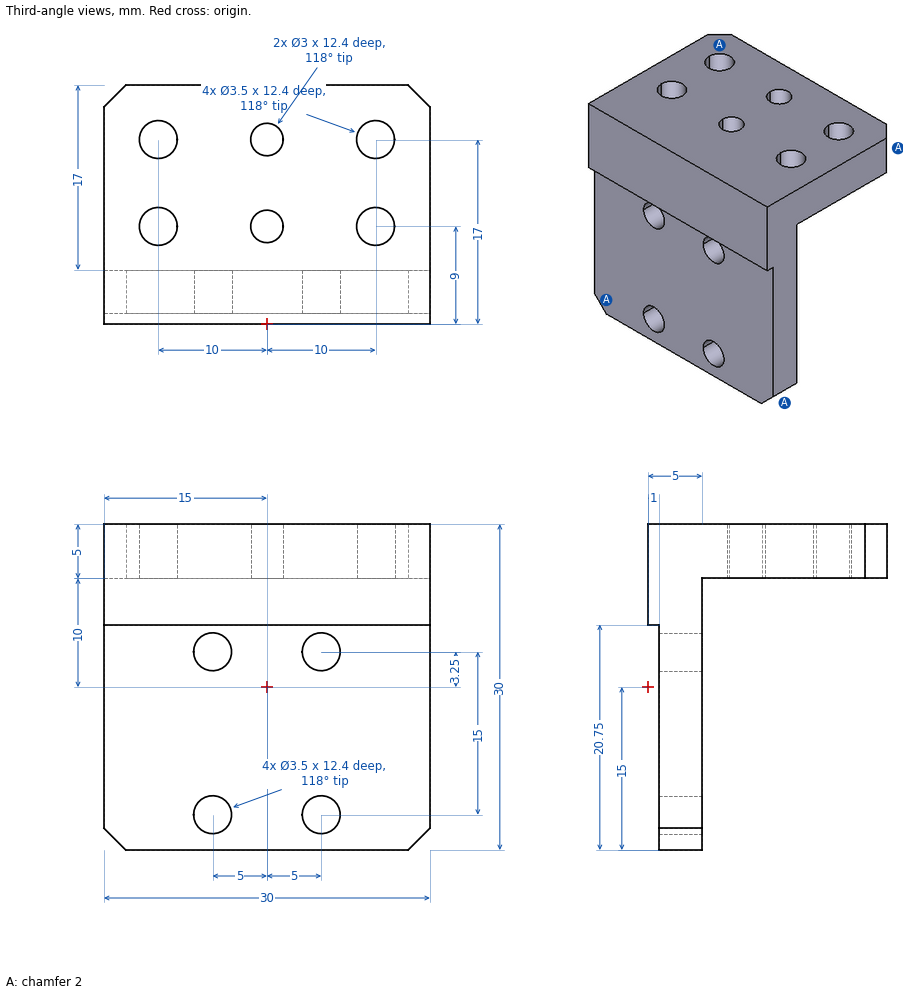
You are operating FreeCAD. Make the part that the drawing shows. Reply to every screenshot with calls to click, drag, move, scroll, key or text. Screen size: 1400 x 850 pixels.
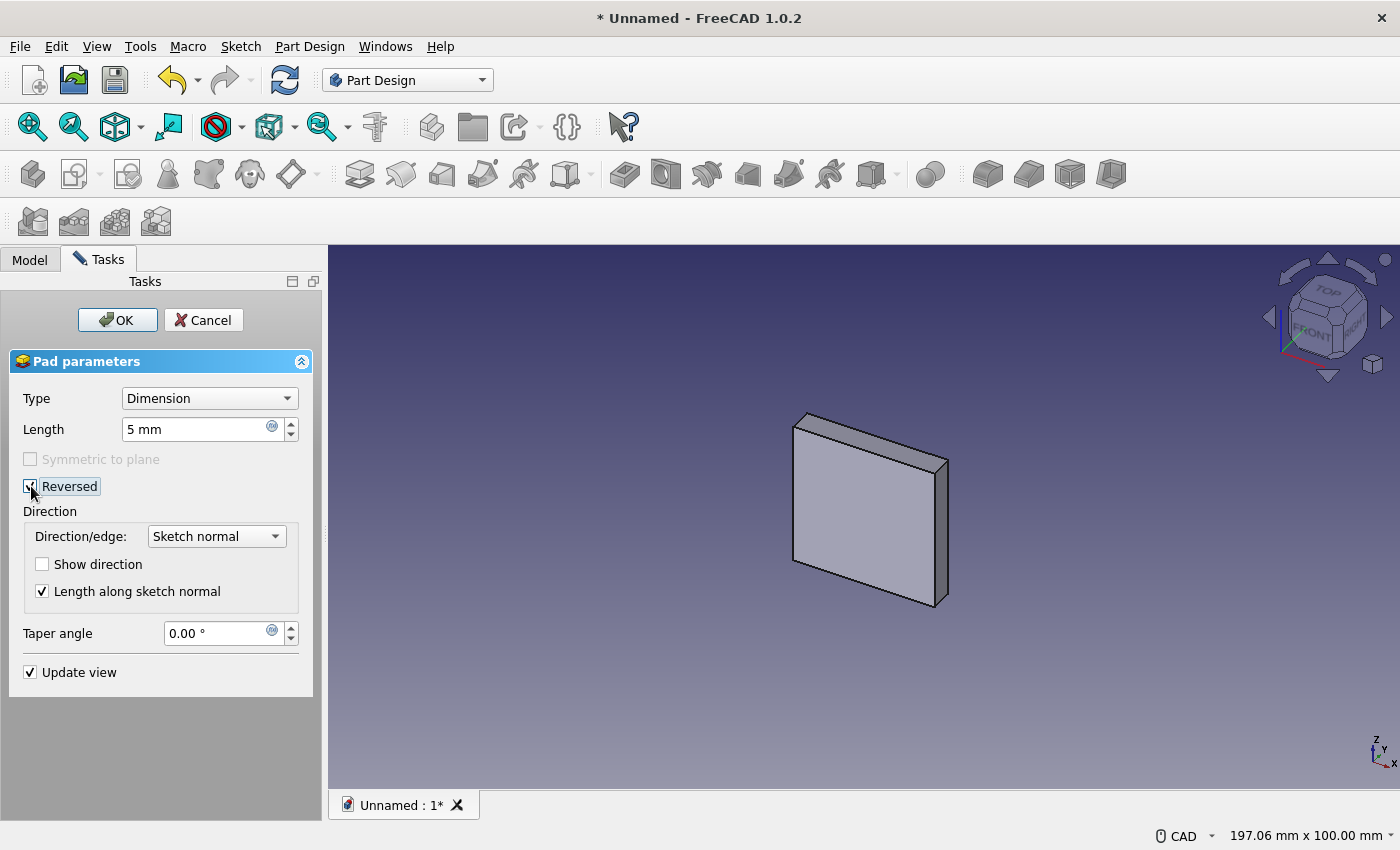
click(118, 320)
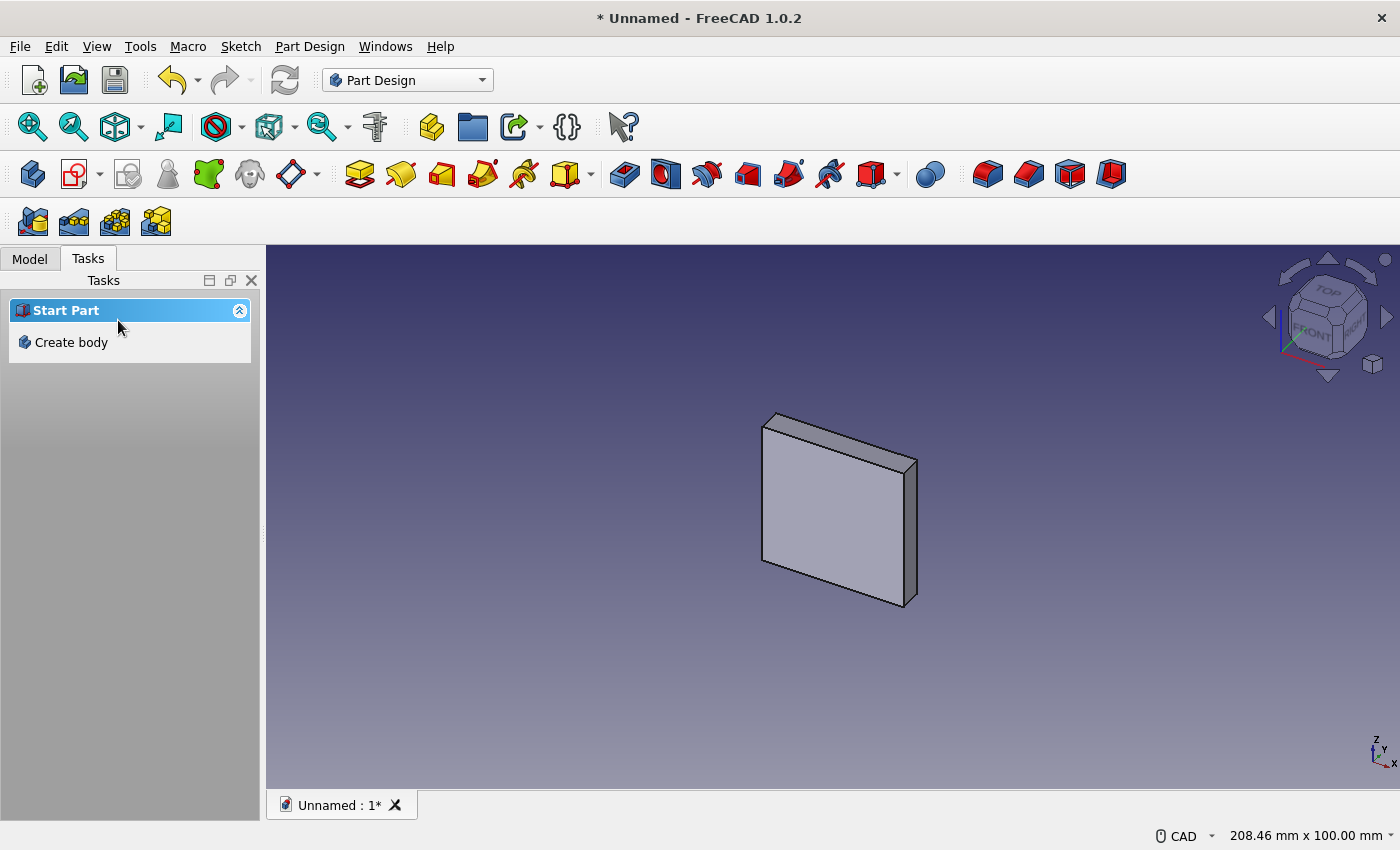
key(v)
key(f)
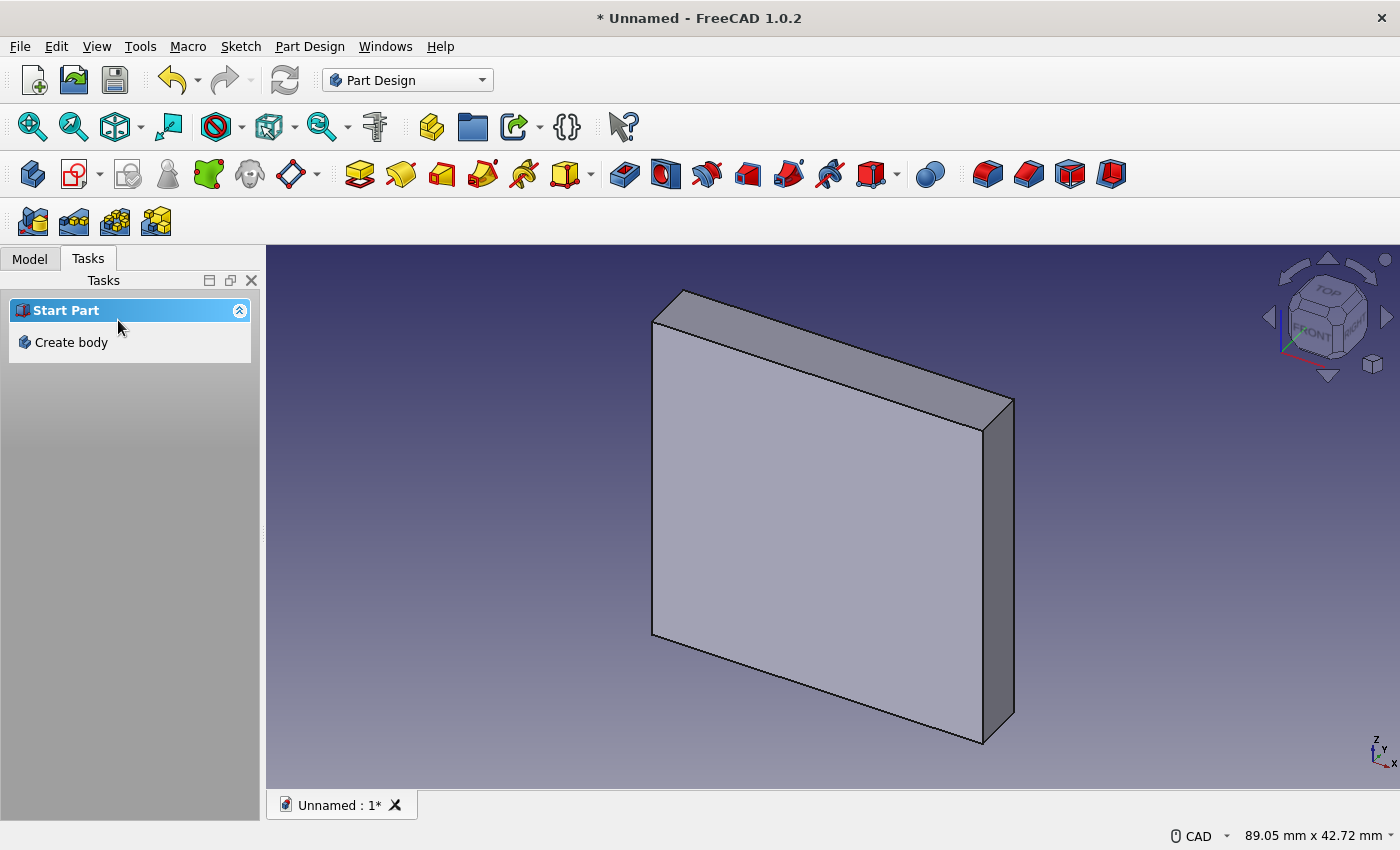
key(4)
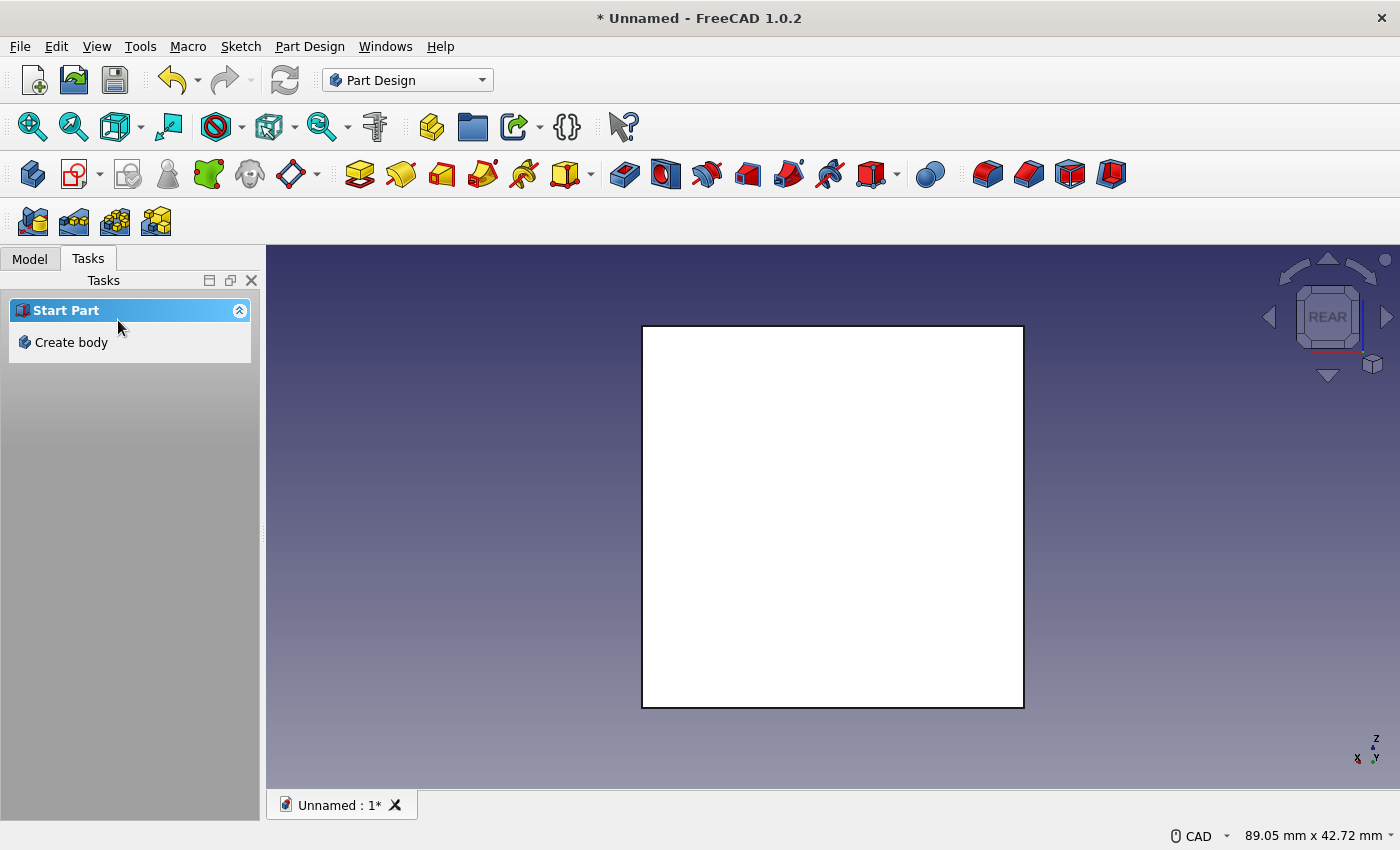
click(833, 516)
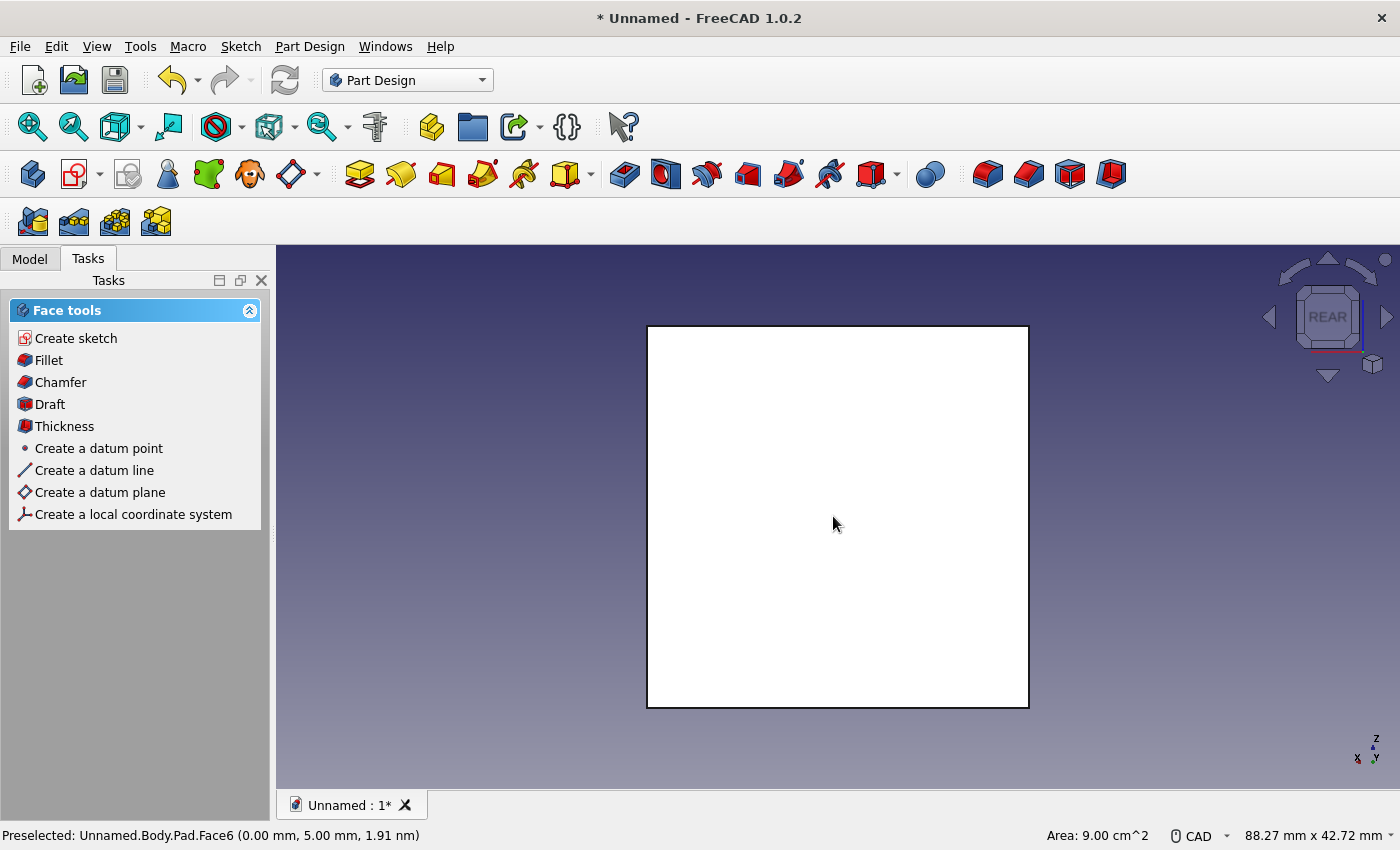
click(74, 174)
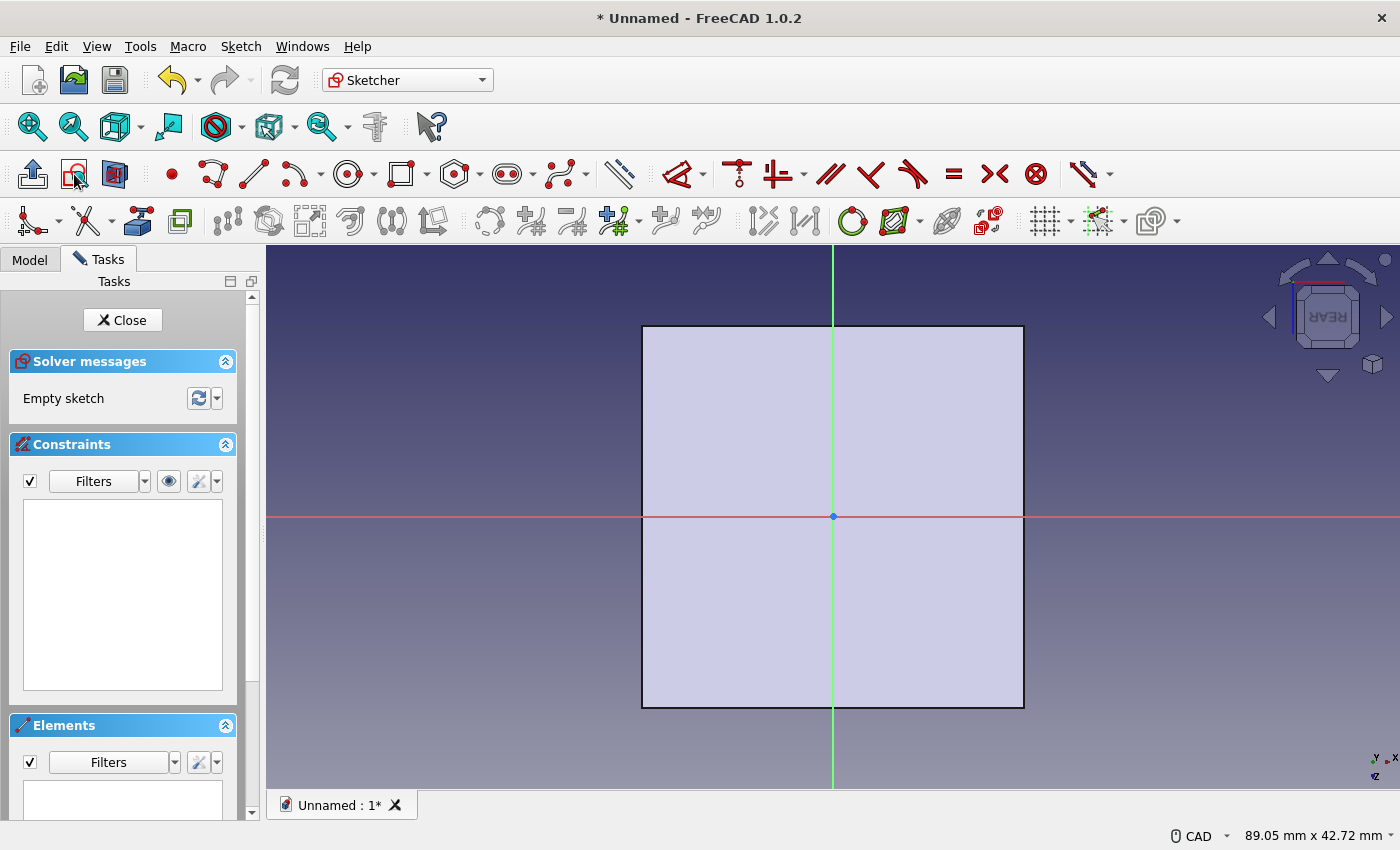
scroll(916, 729, up, 3)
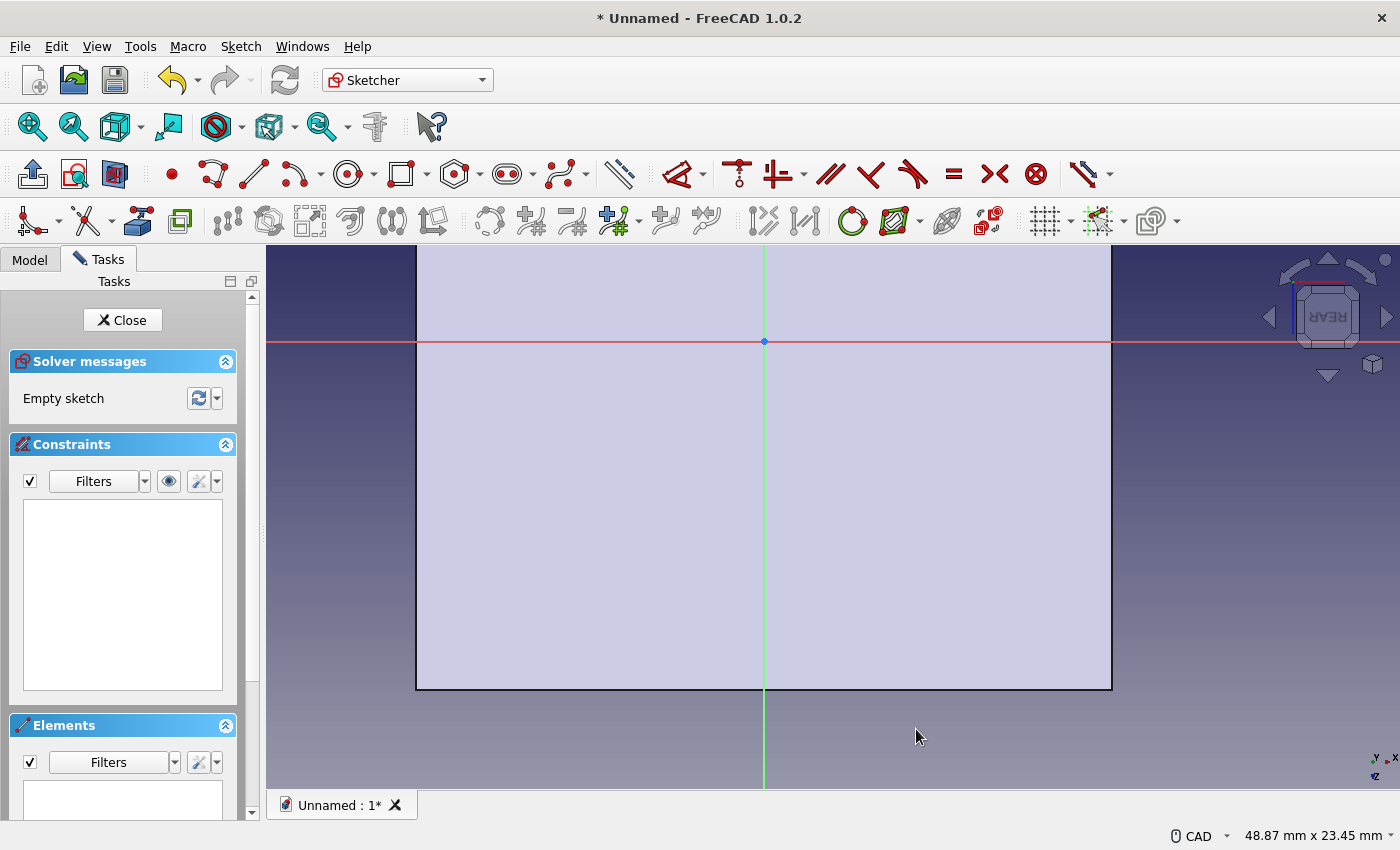
key(g)
key(r)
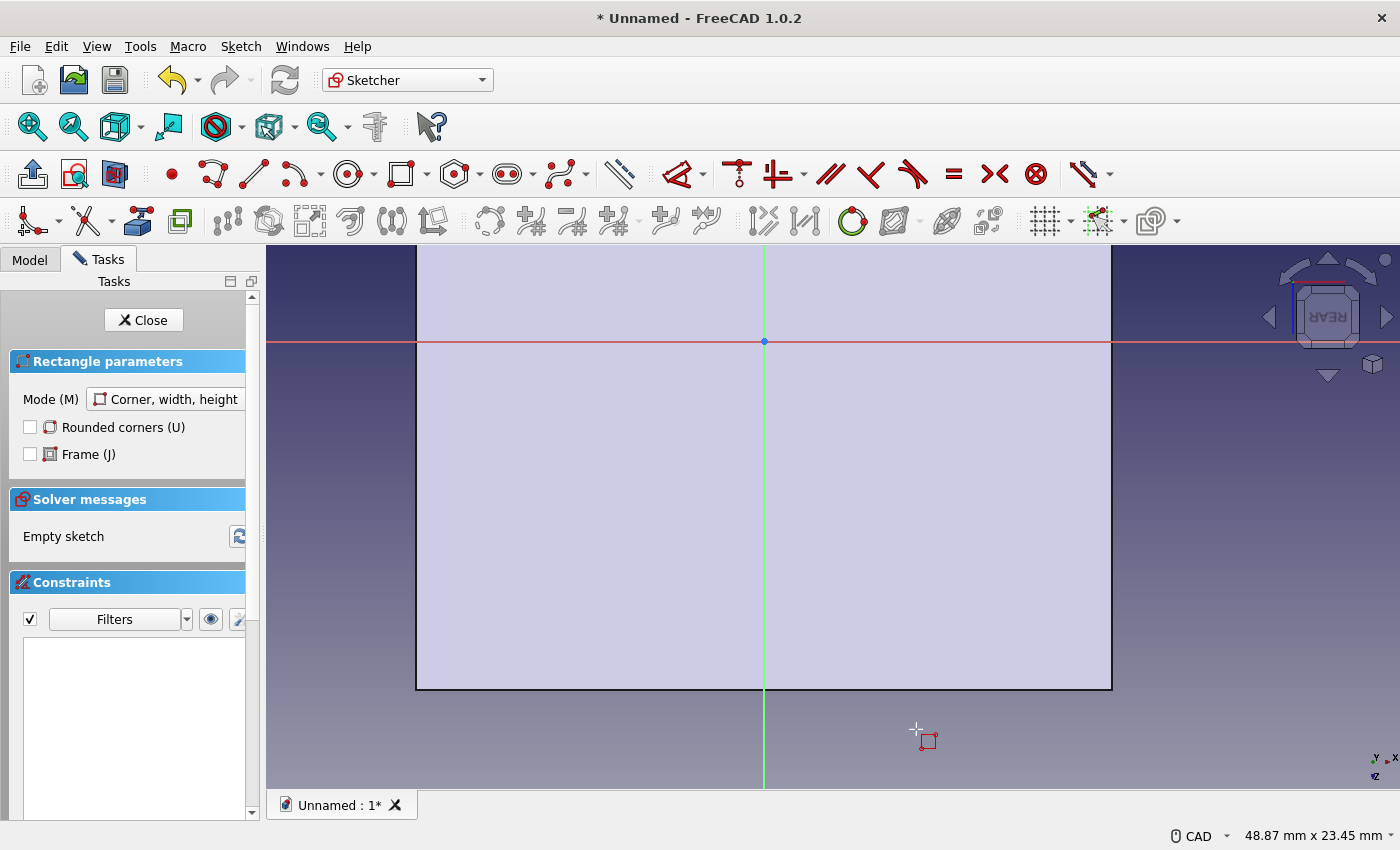
click(416, 574)
click(1112, 690)
key(Escape)